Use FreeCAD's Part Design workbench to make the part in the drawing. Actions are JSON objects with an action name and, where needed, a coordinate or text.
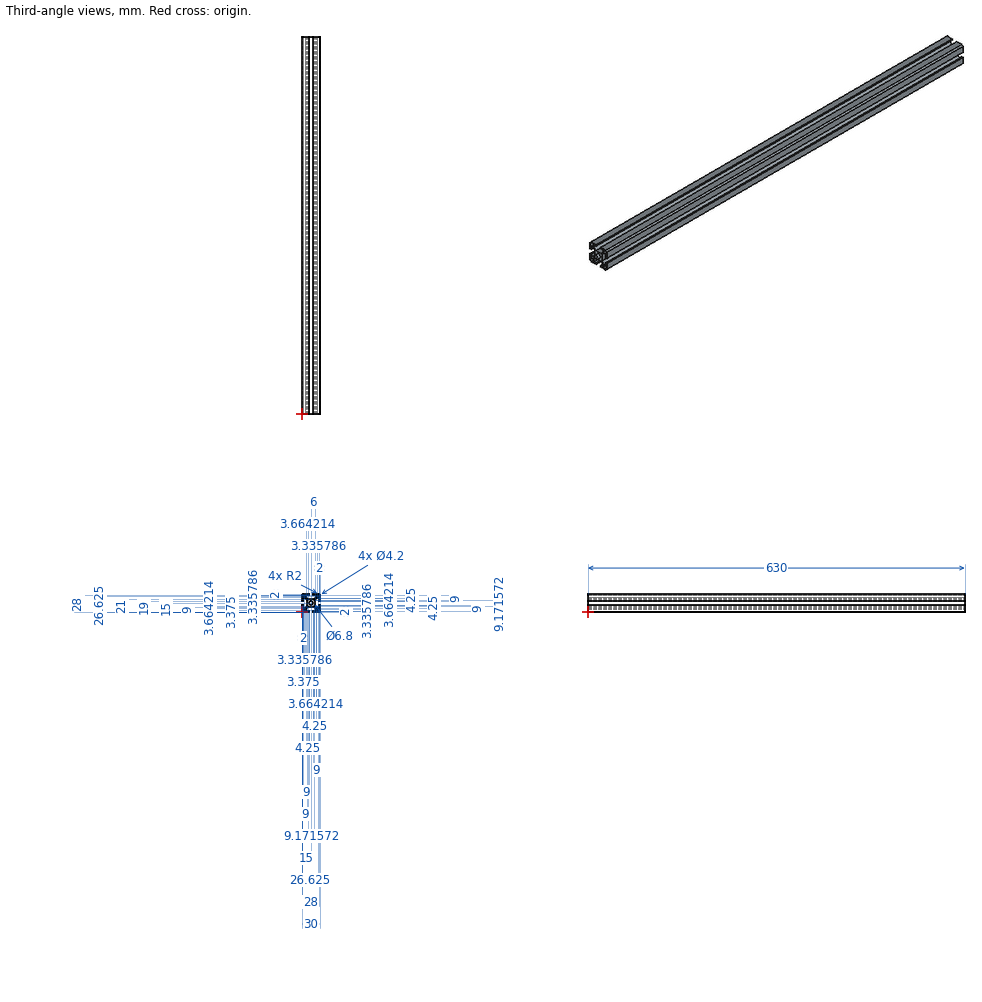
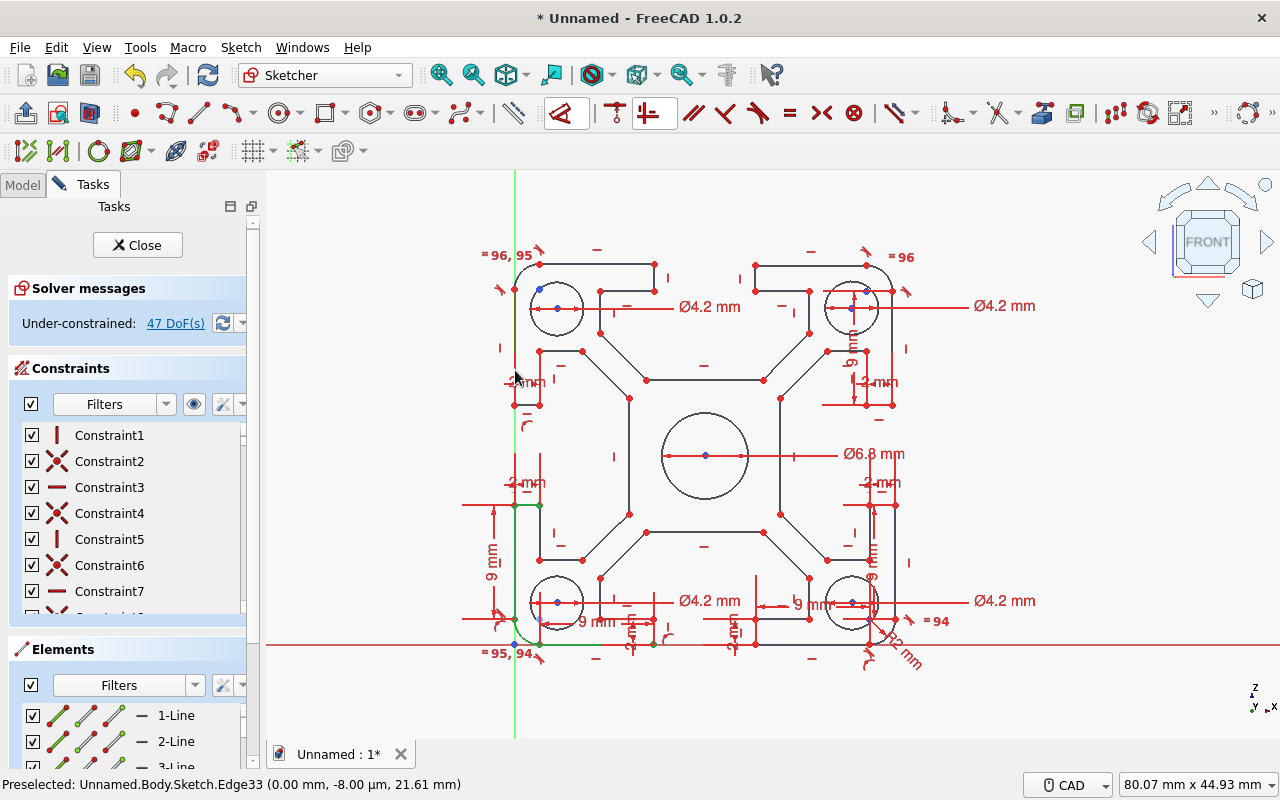
{"action": "left_click", "coordinate": [584, 114]}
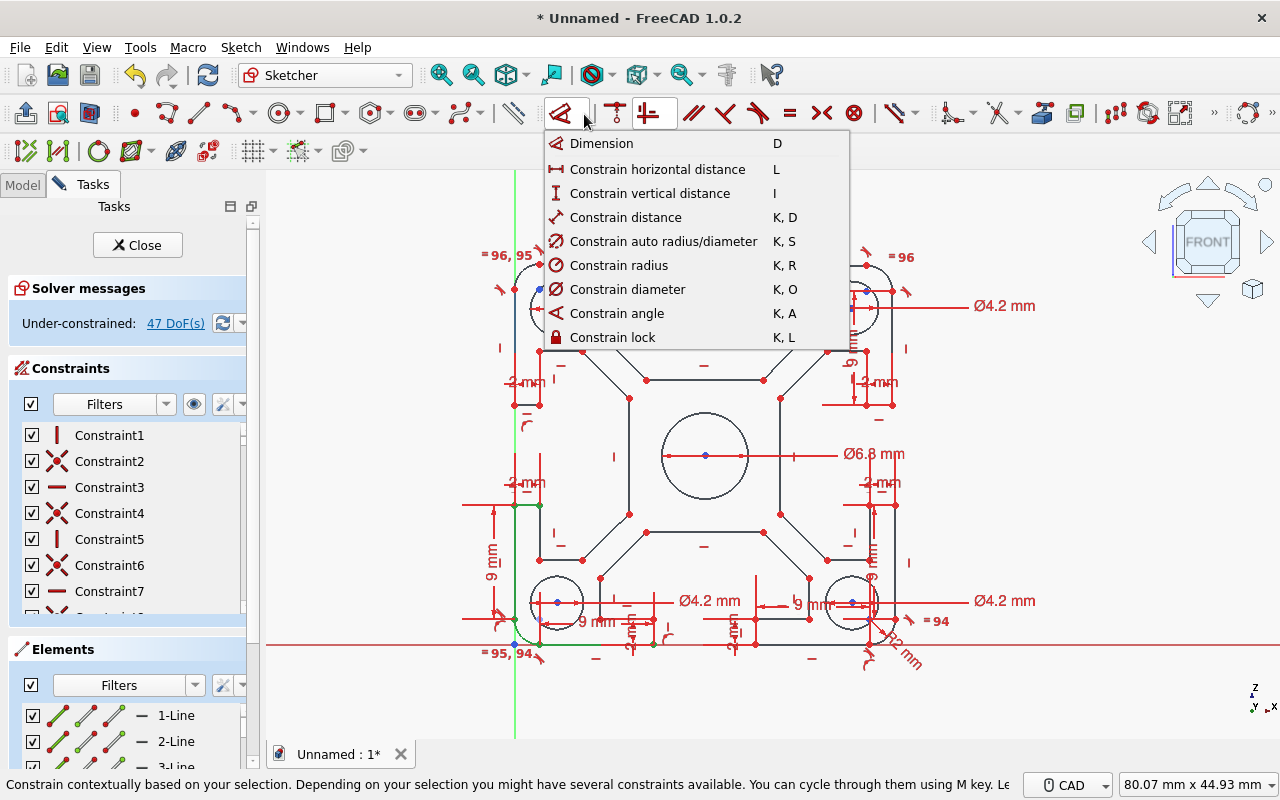
{"action": "left_click", "coordinate": [697, 193]}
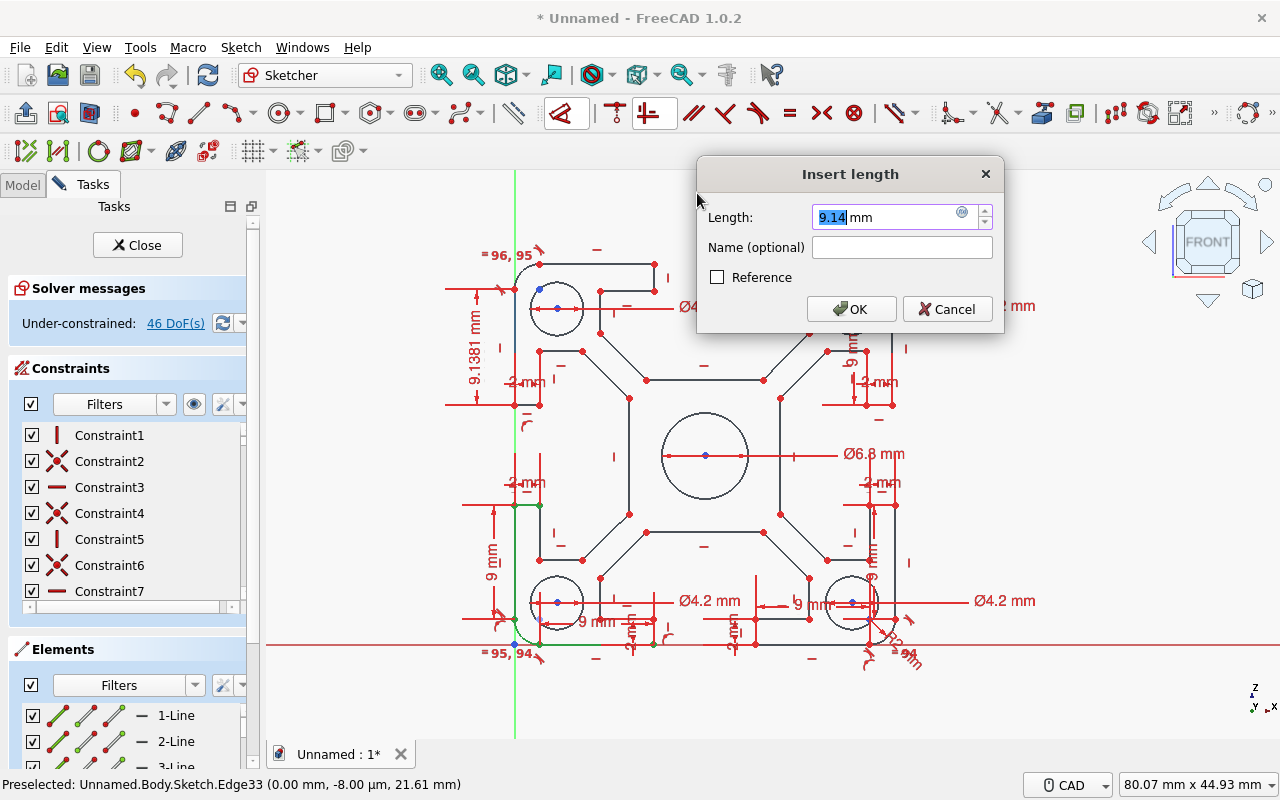
{"action": "type", "text": "9"}
{"action": "key", "text": "Return"}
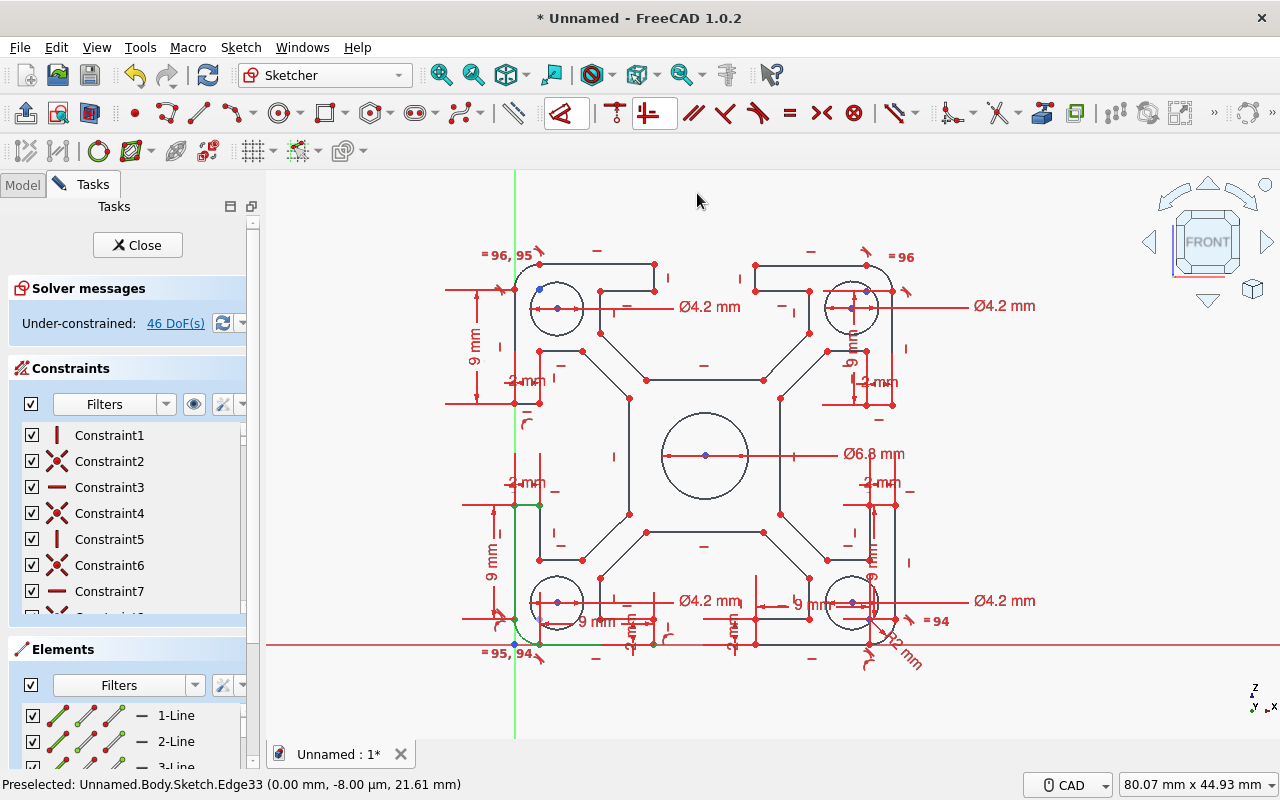
{"action": "left_click", "coordinate": [574, 264]}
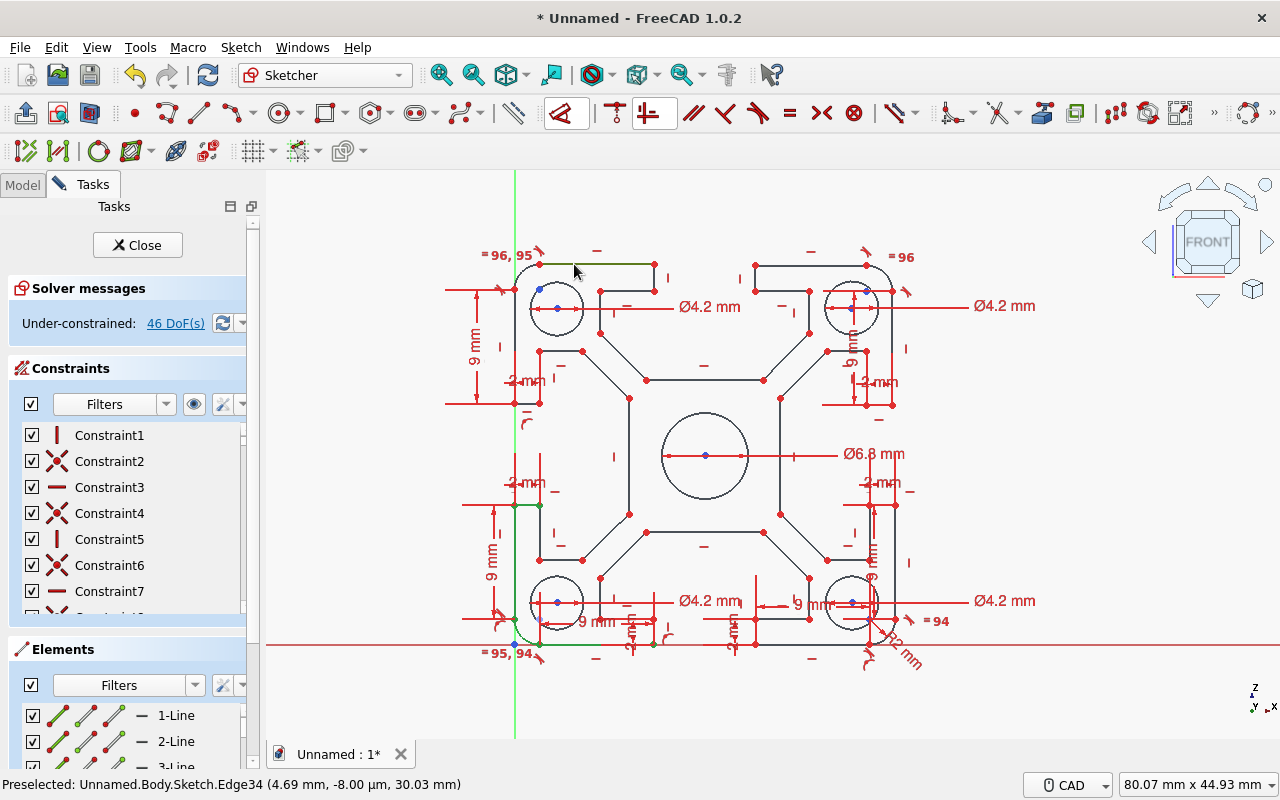
{"action": "left_click", "coordinate": [584, 114]}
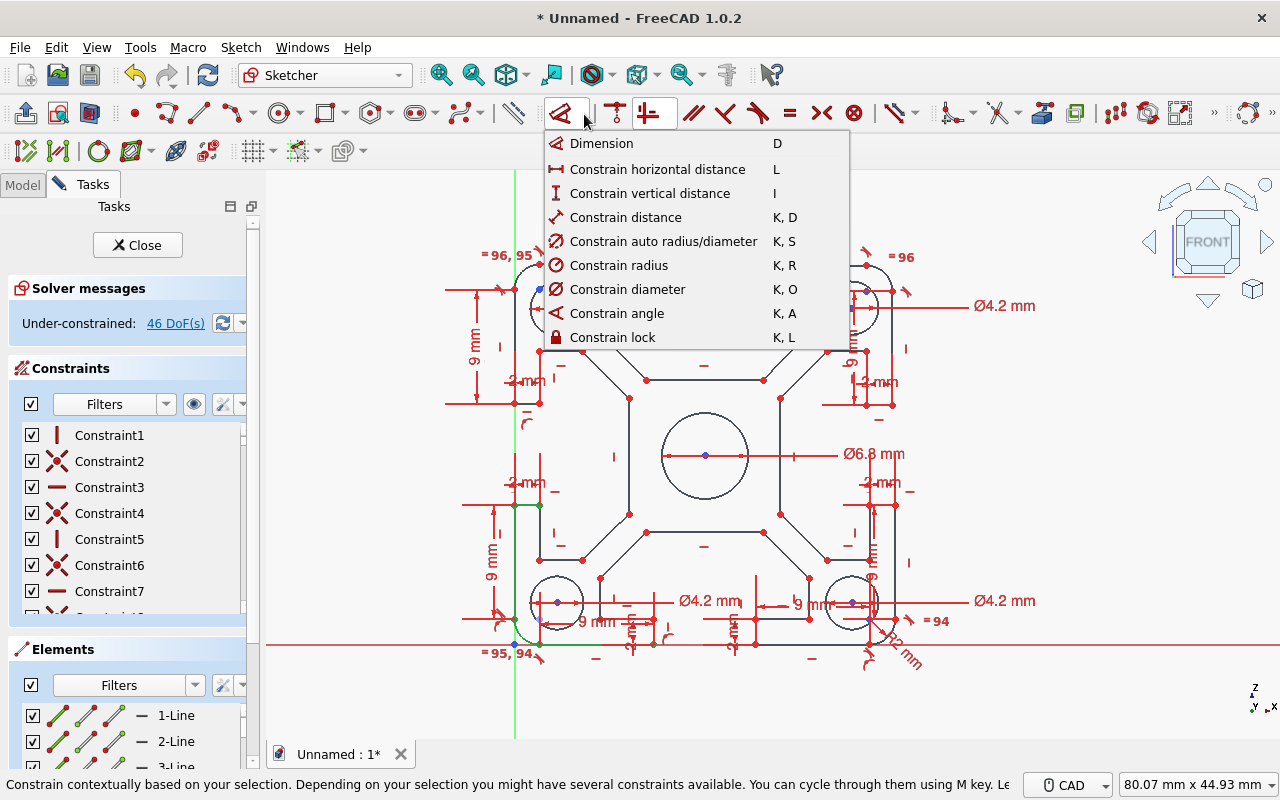
{"action": "left_click", "coordinate": [697, 169]}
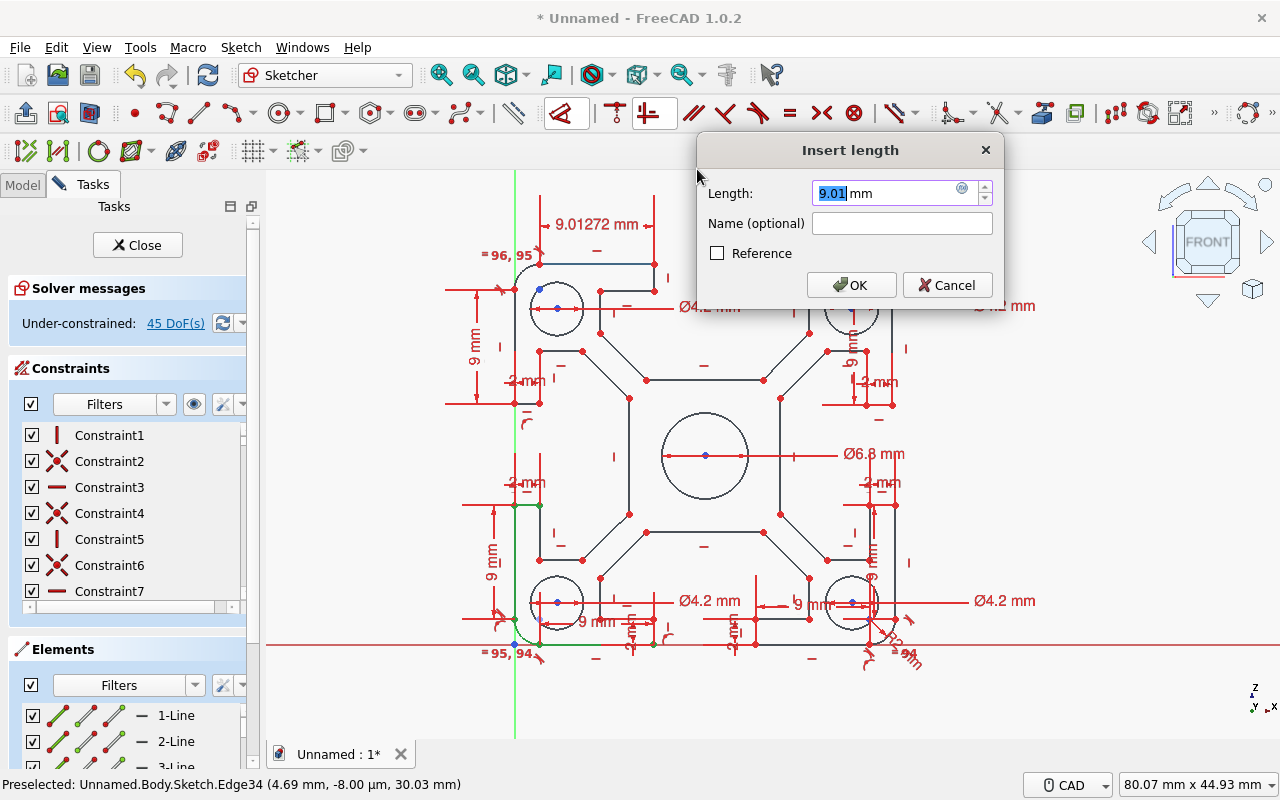
{"action": "type", "text": "9"}
{"action": "key", "text": "Return"}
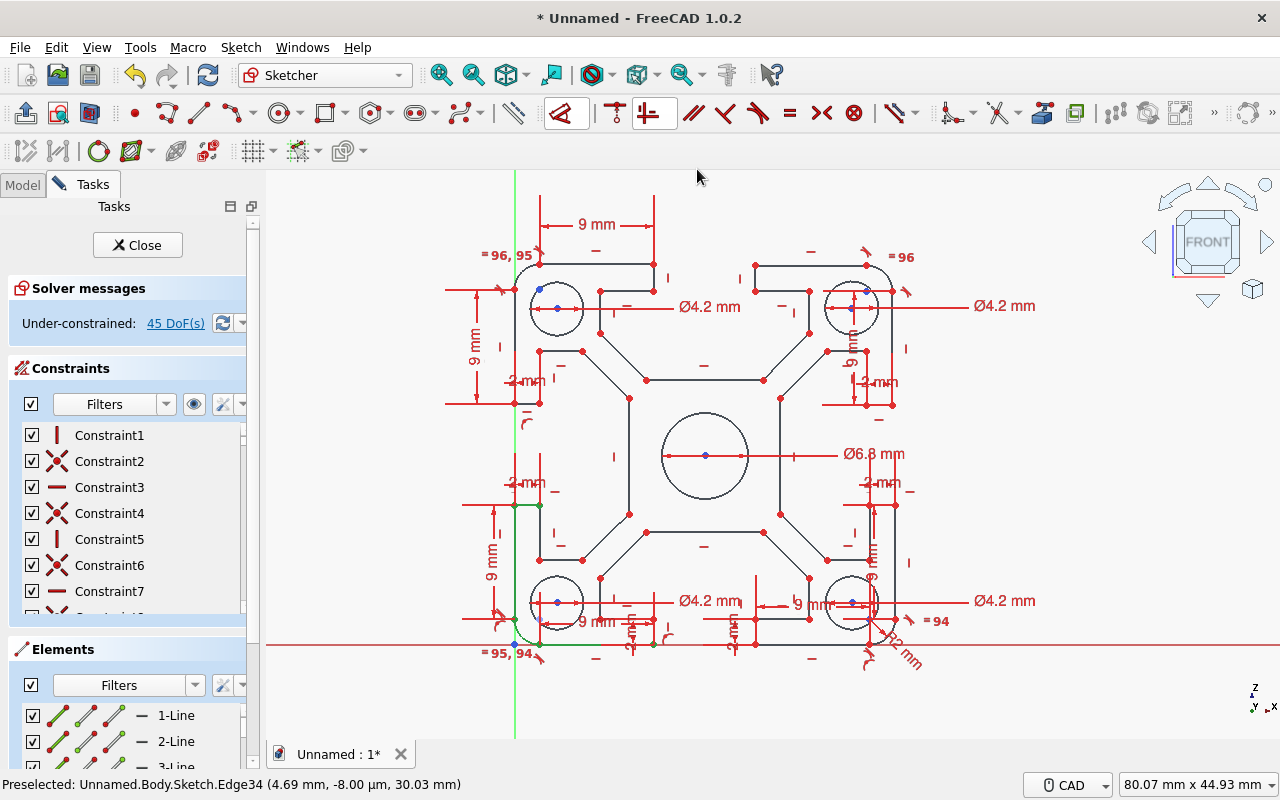
{"action": "scroll", "coordinate": [654, 275], "scroll_direction": "up", "scroll_amount": 3}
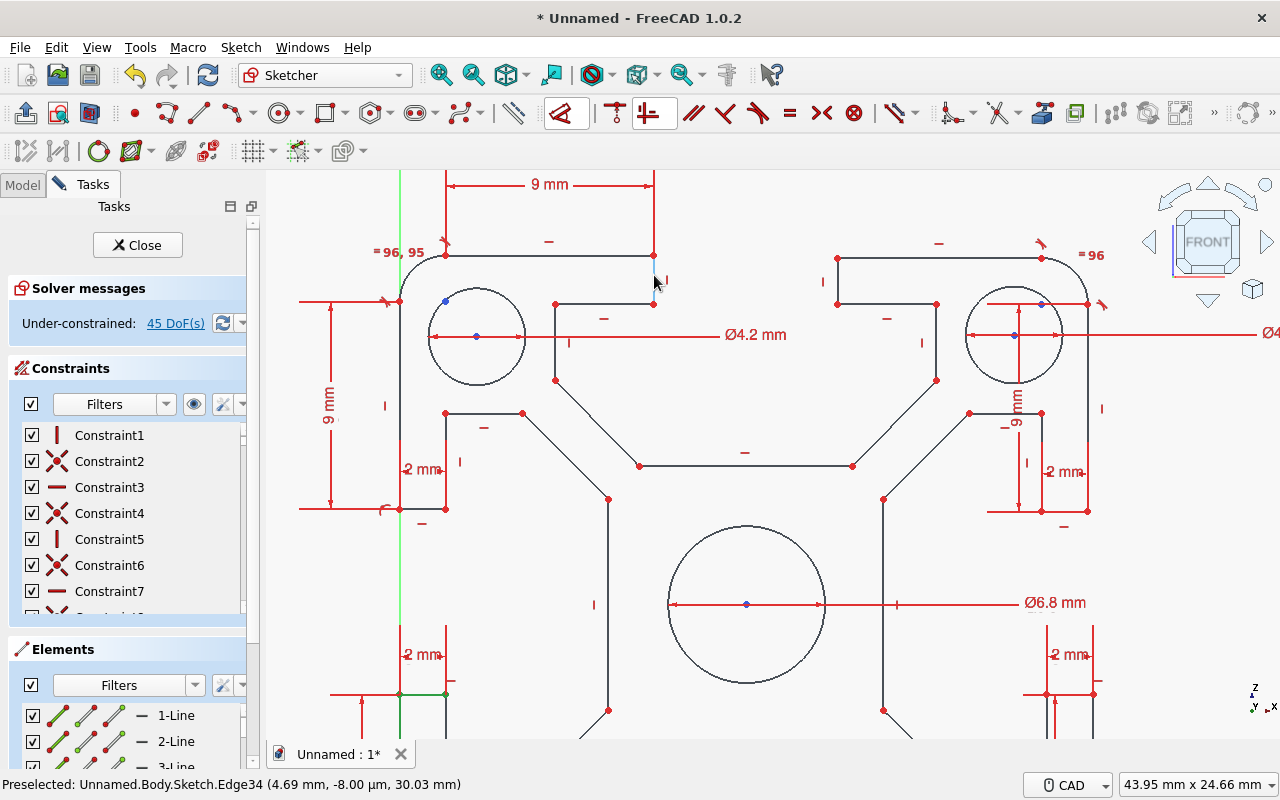
{"action": "left_click", "coordinate": [654, 275]}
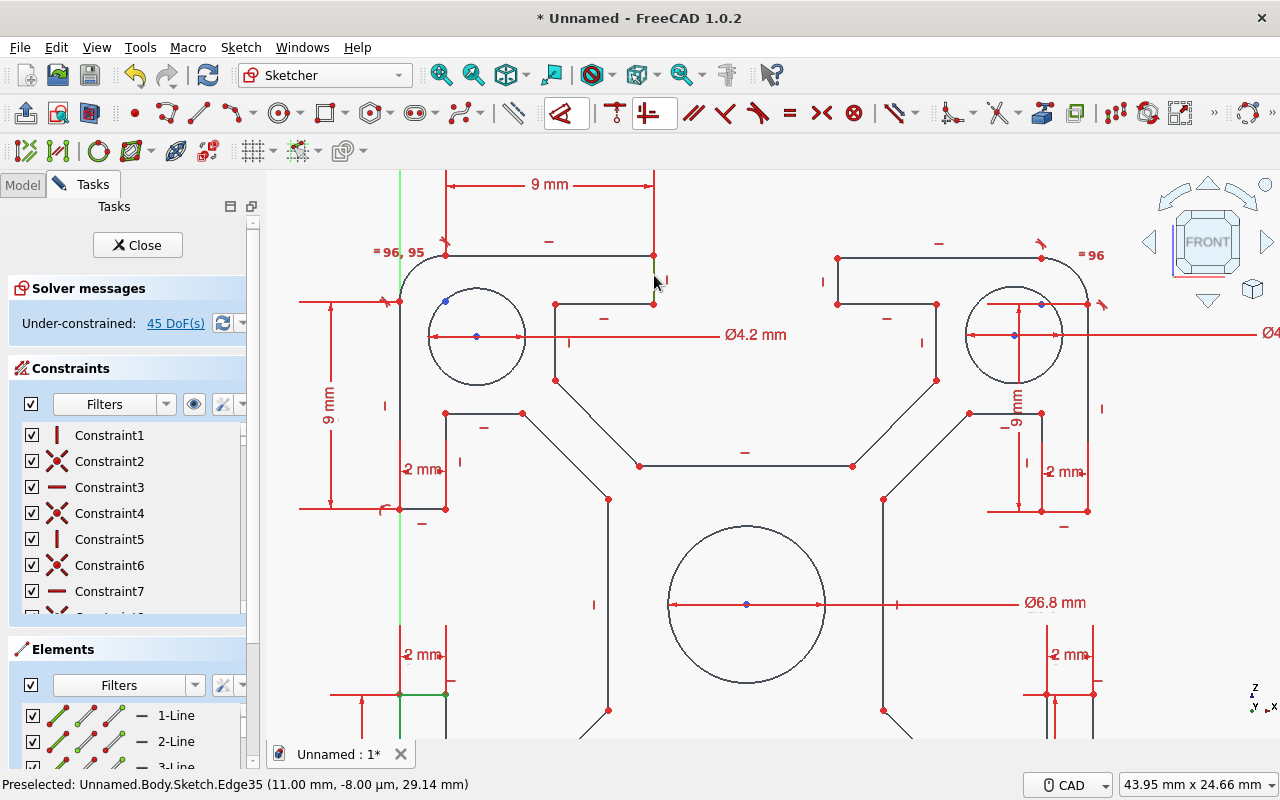
{"action": "left_click", "coordinate": [584, 114]}